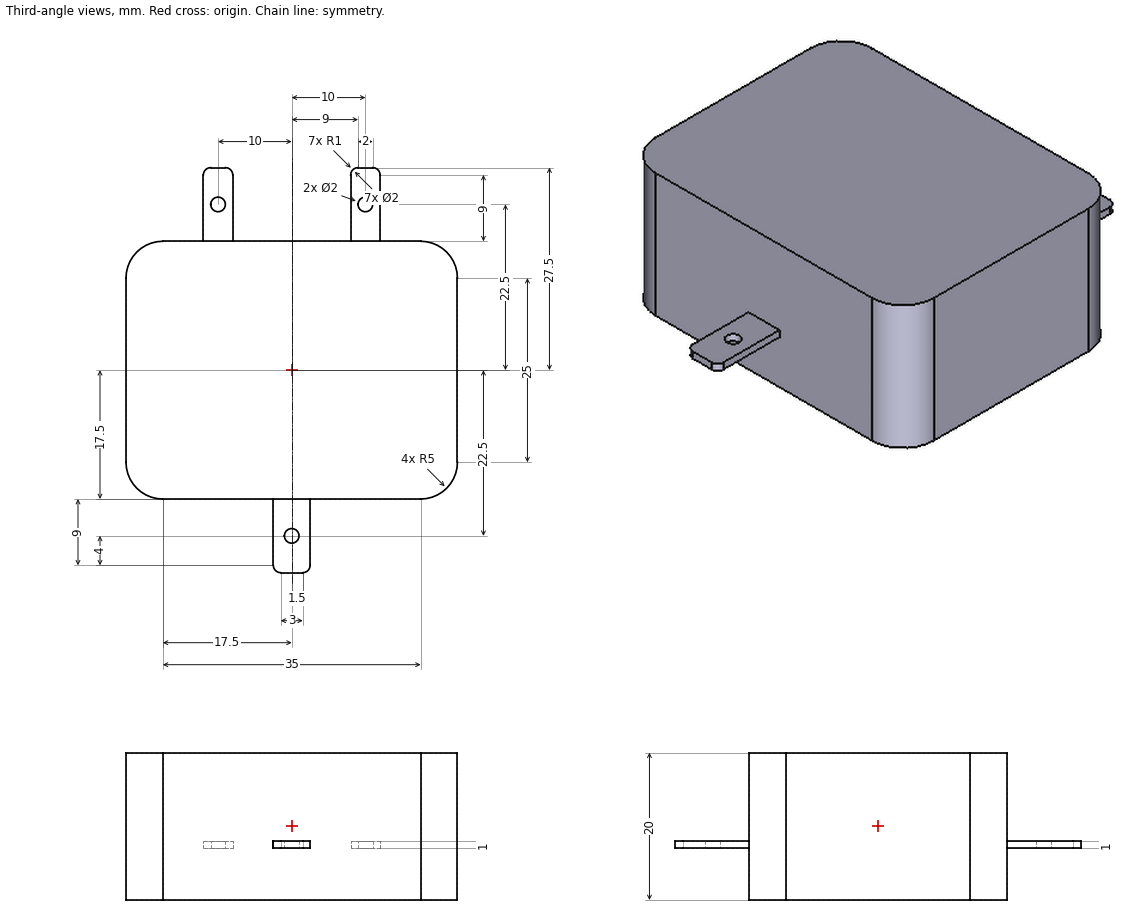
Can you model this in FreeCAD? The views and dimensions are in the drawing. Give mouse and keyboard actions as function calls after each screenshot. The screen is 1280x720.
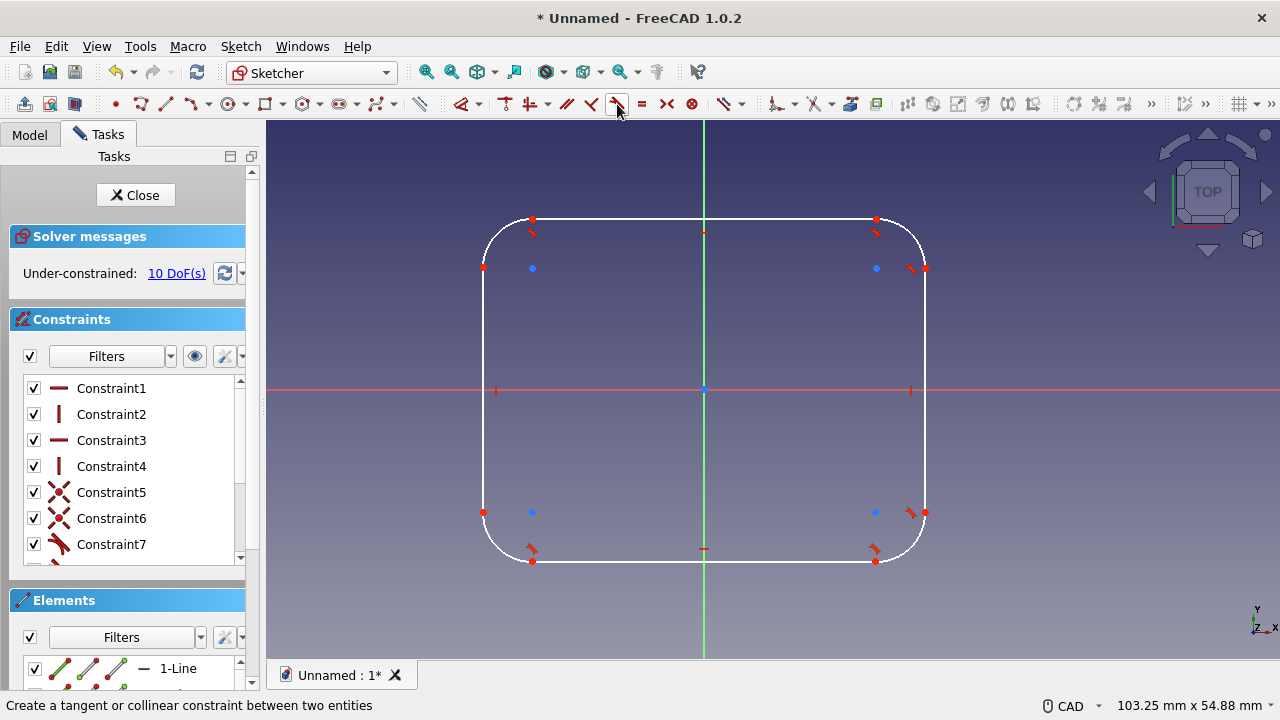
click(483, 342)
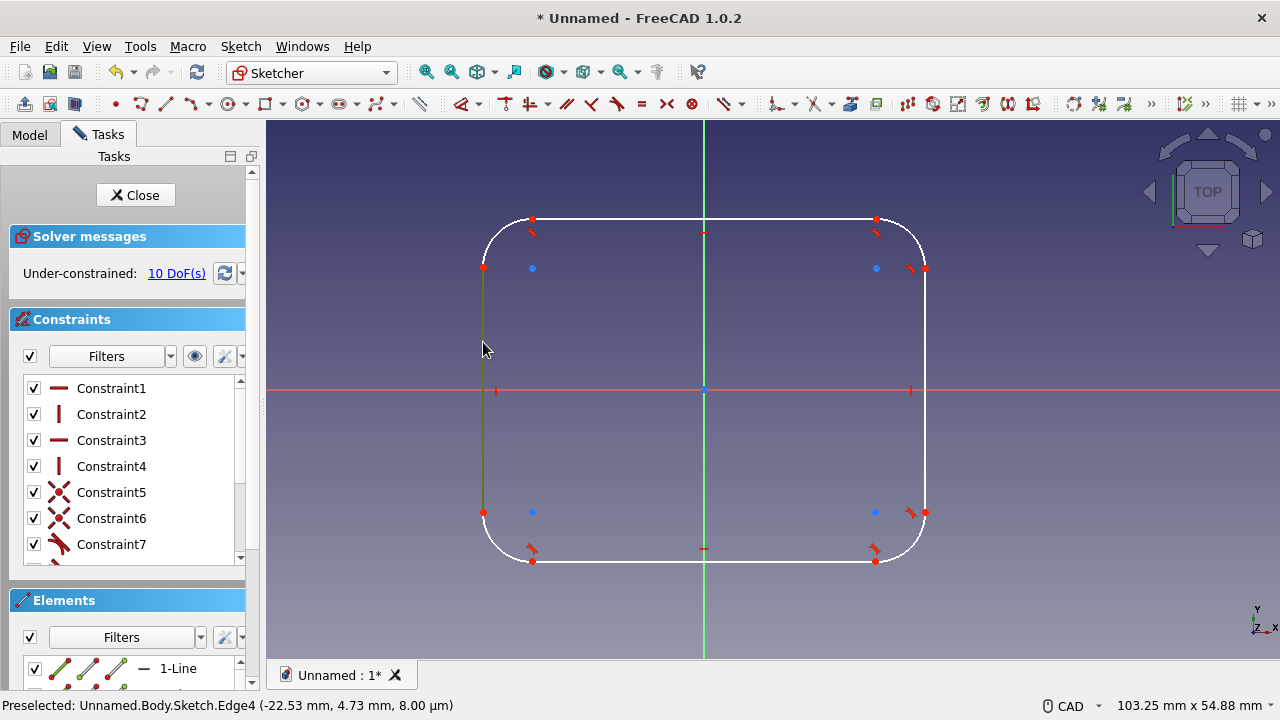
click(510, 224)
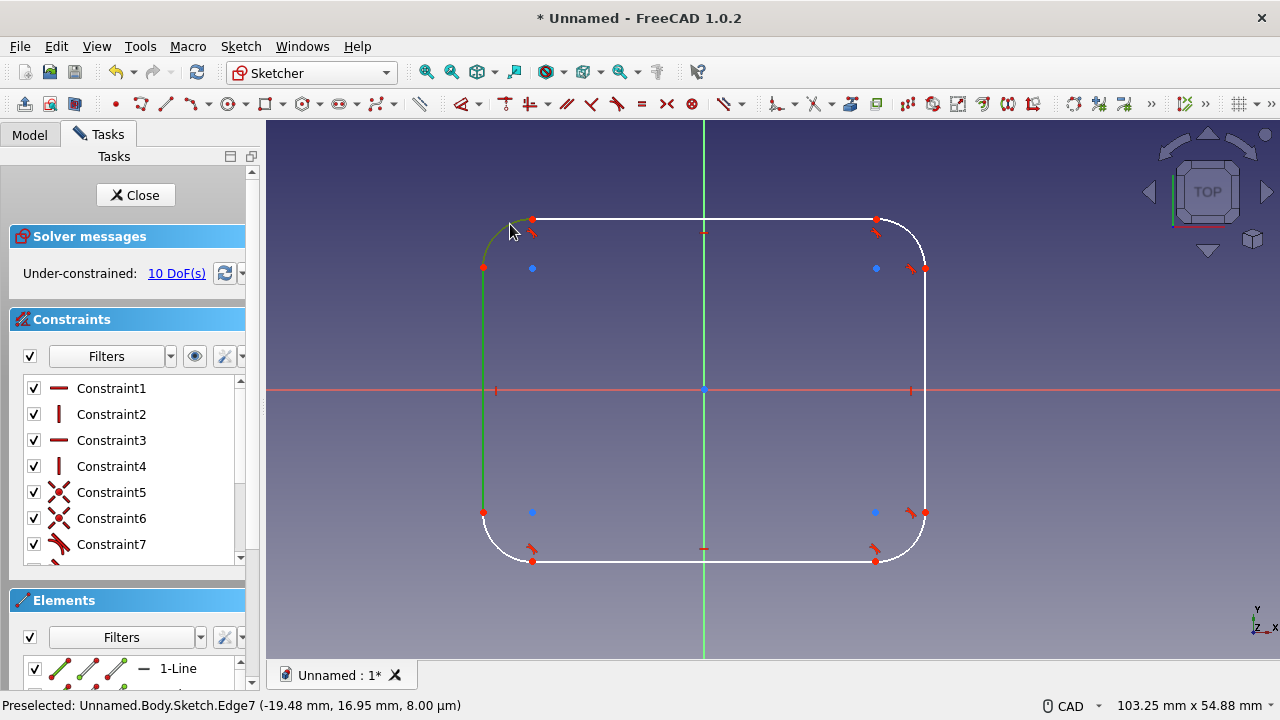
click(617, 104)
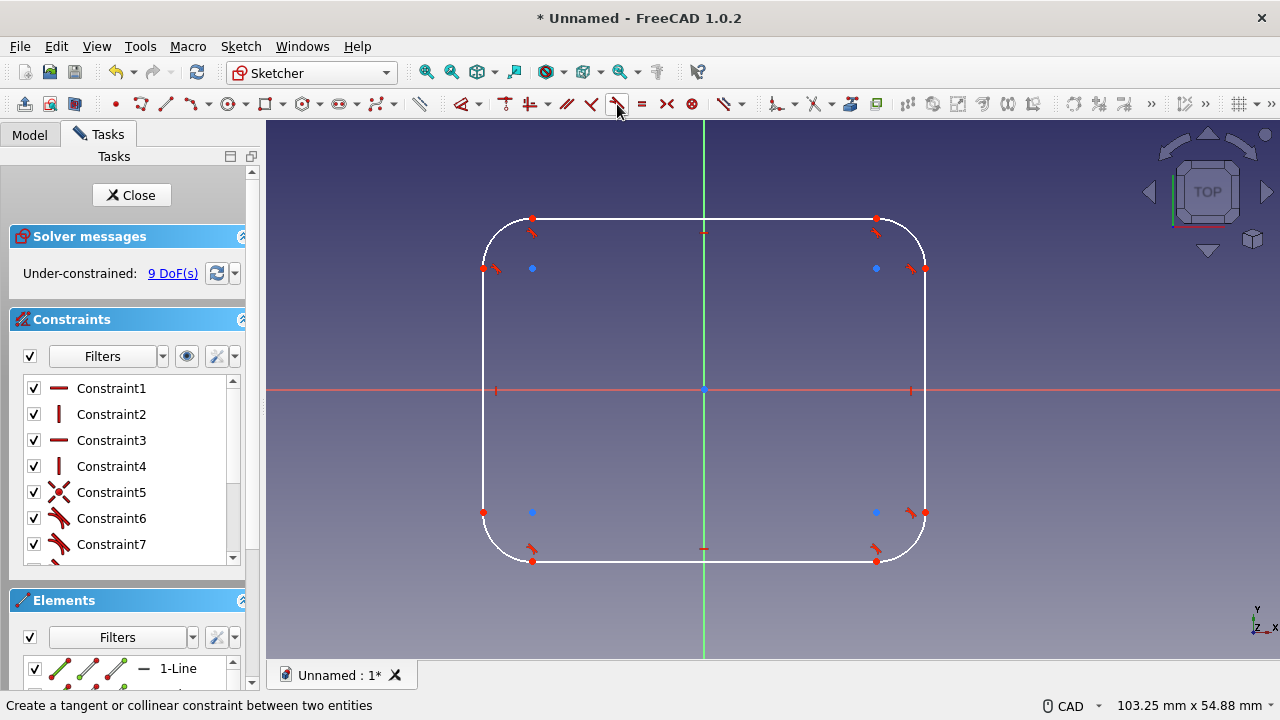
click(483, 342)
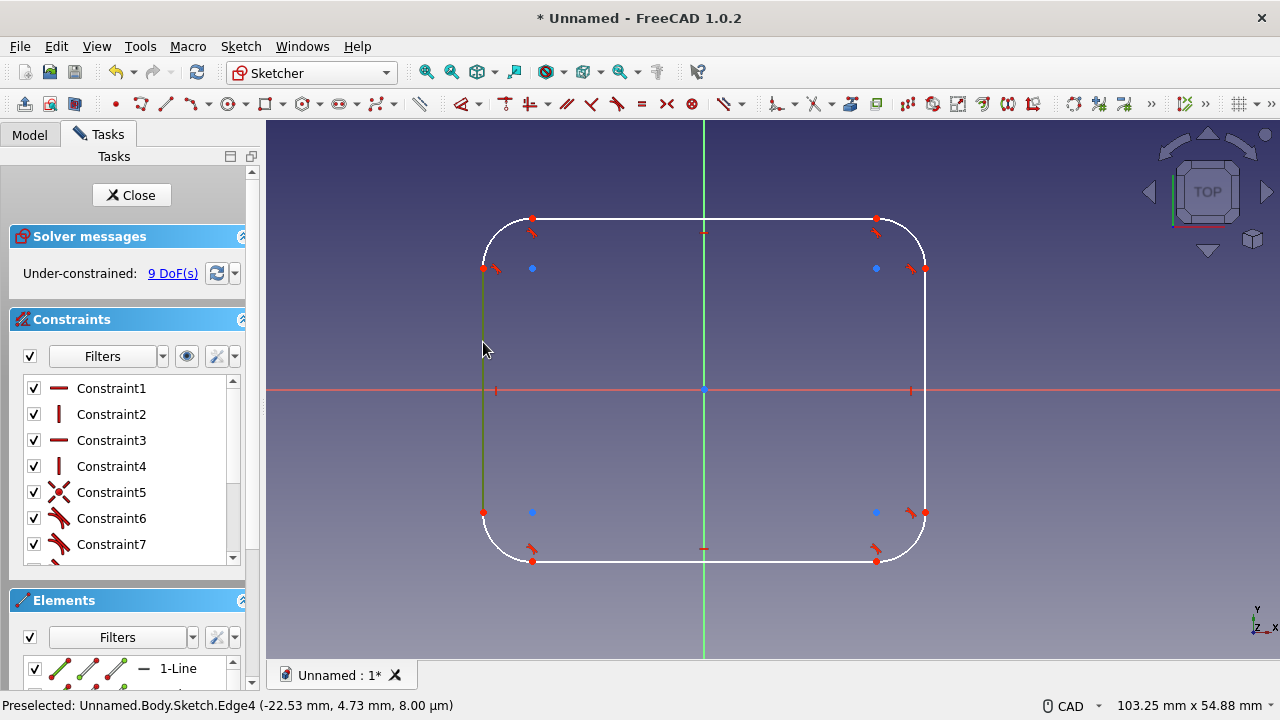
click(489, 535)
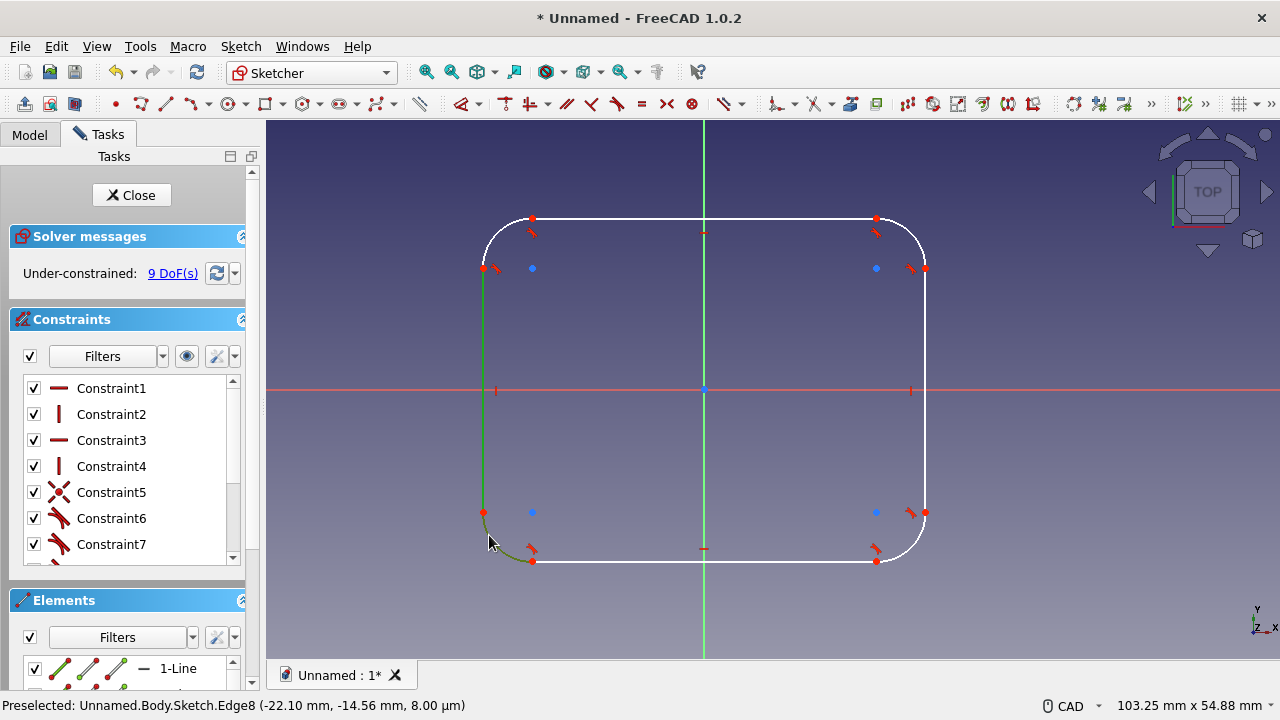
key(t)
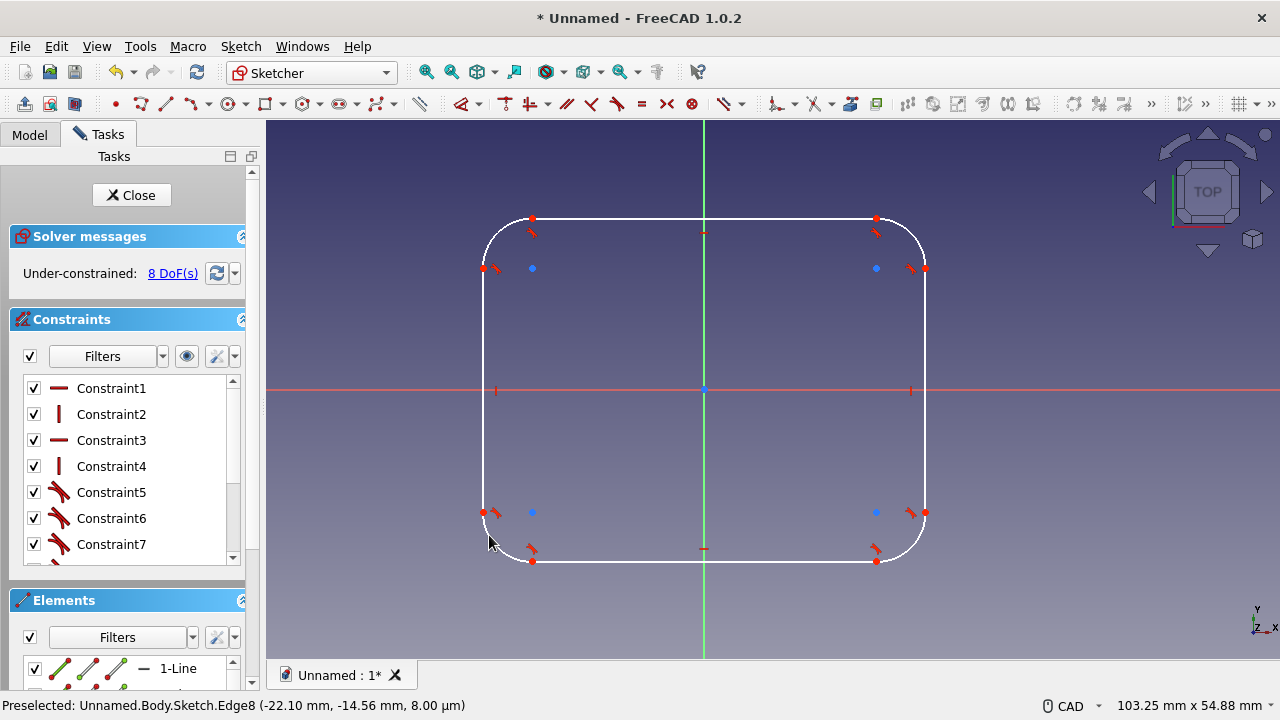
click(899, 557)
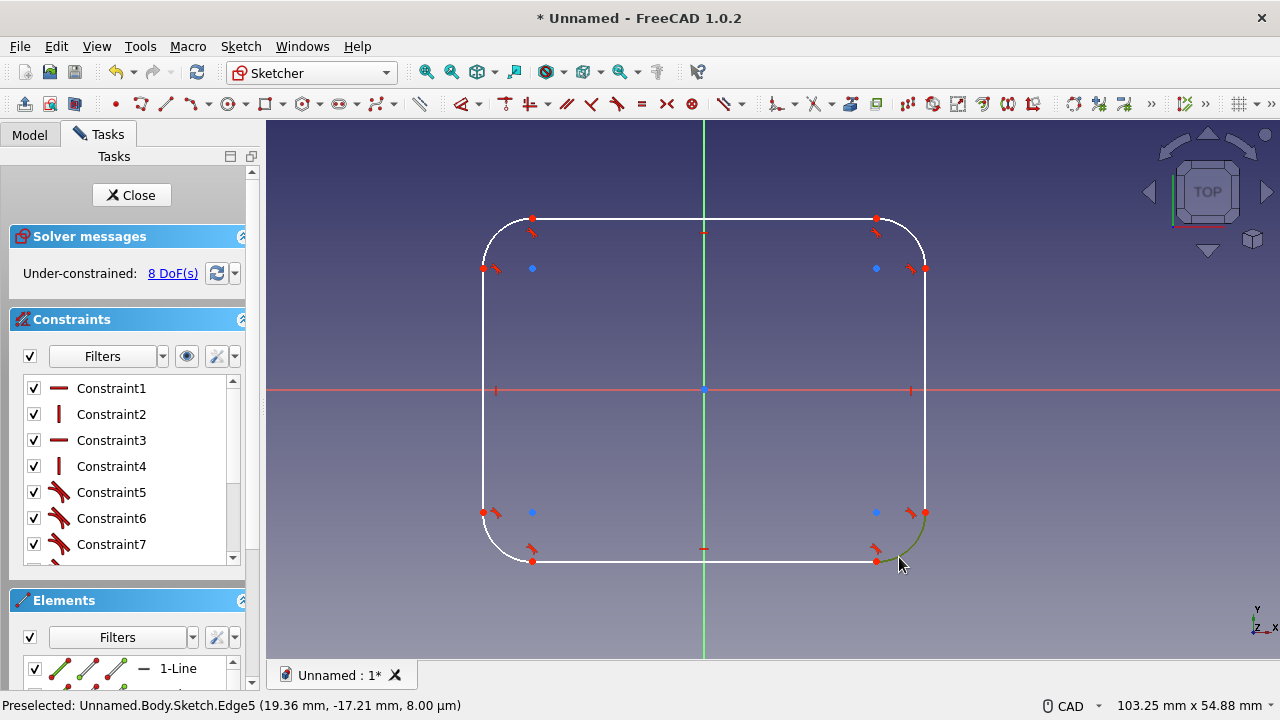
click(920, 246)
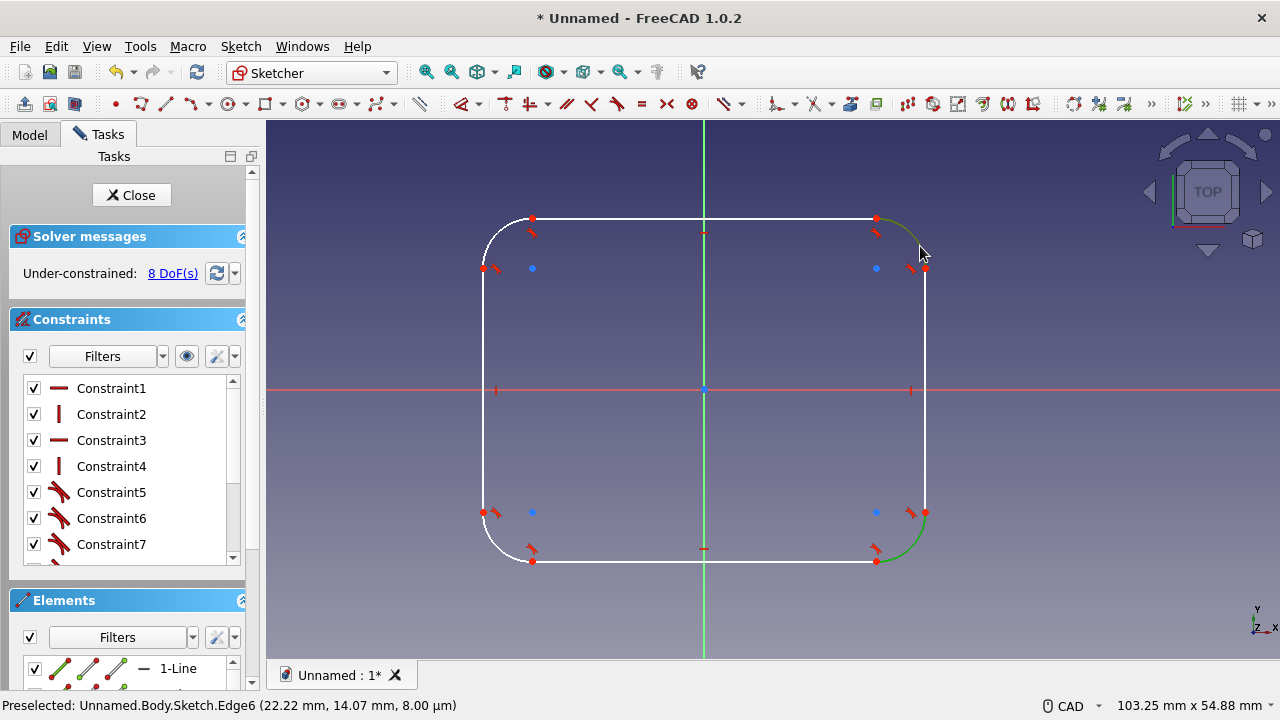
click(510, 224)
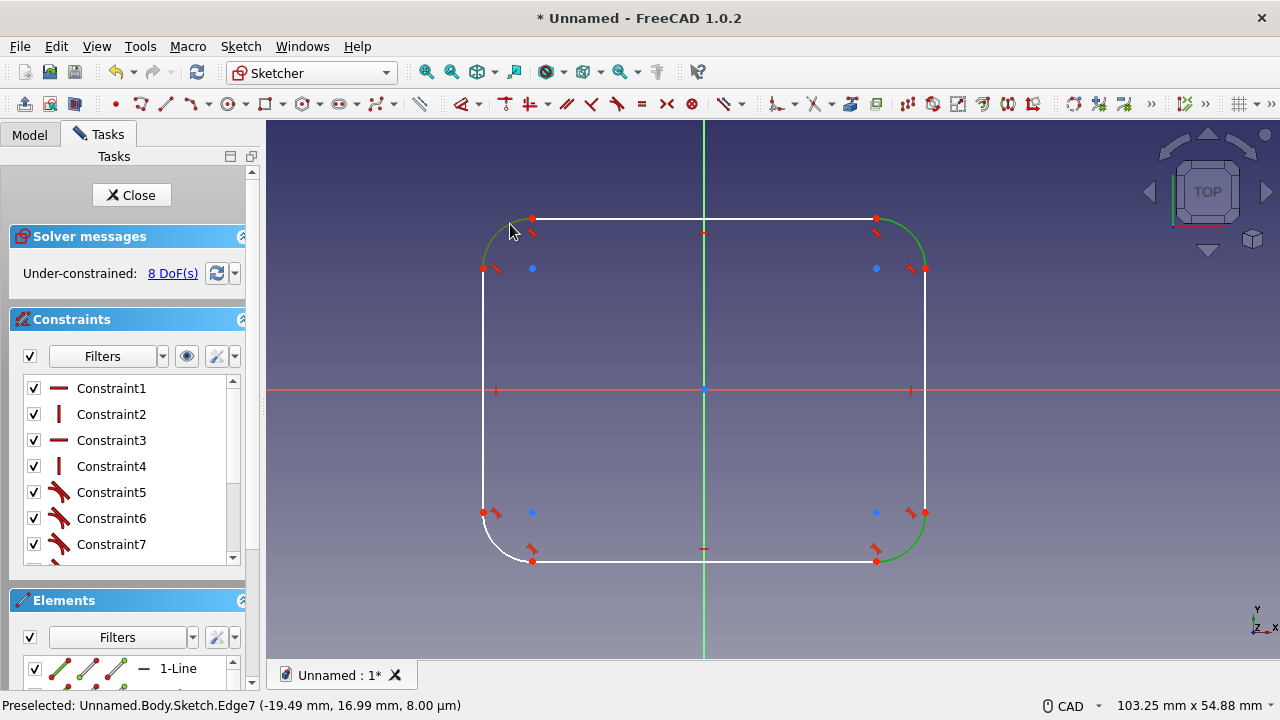
click(488, 535)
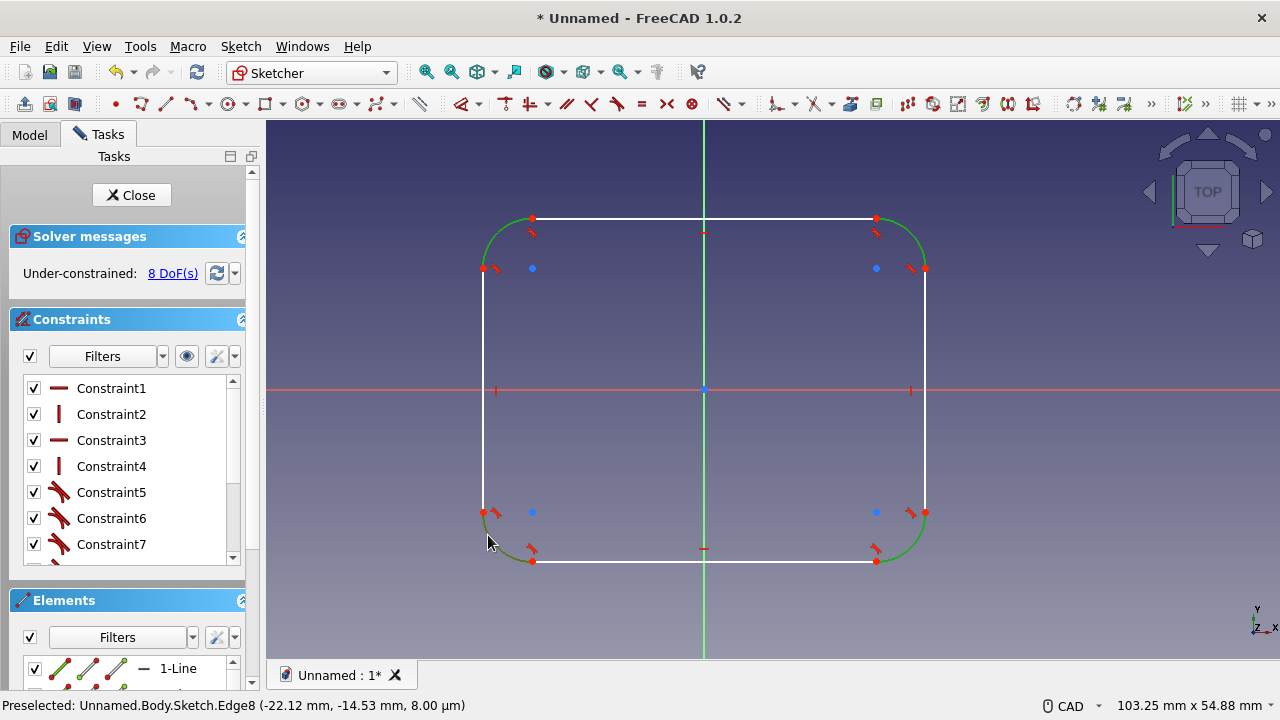
click(642, 104)